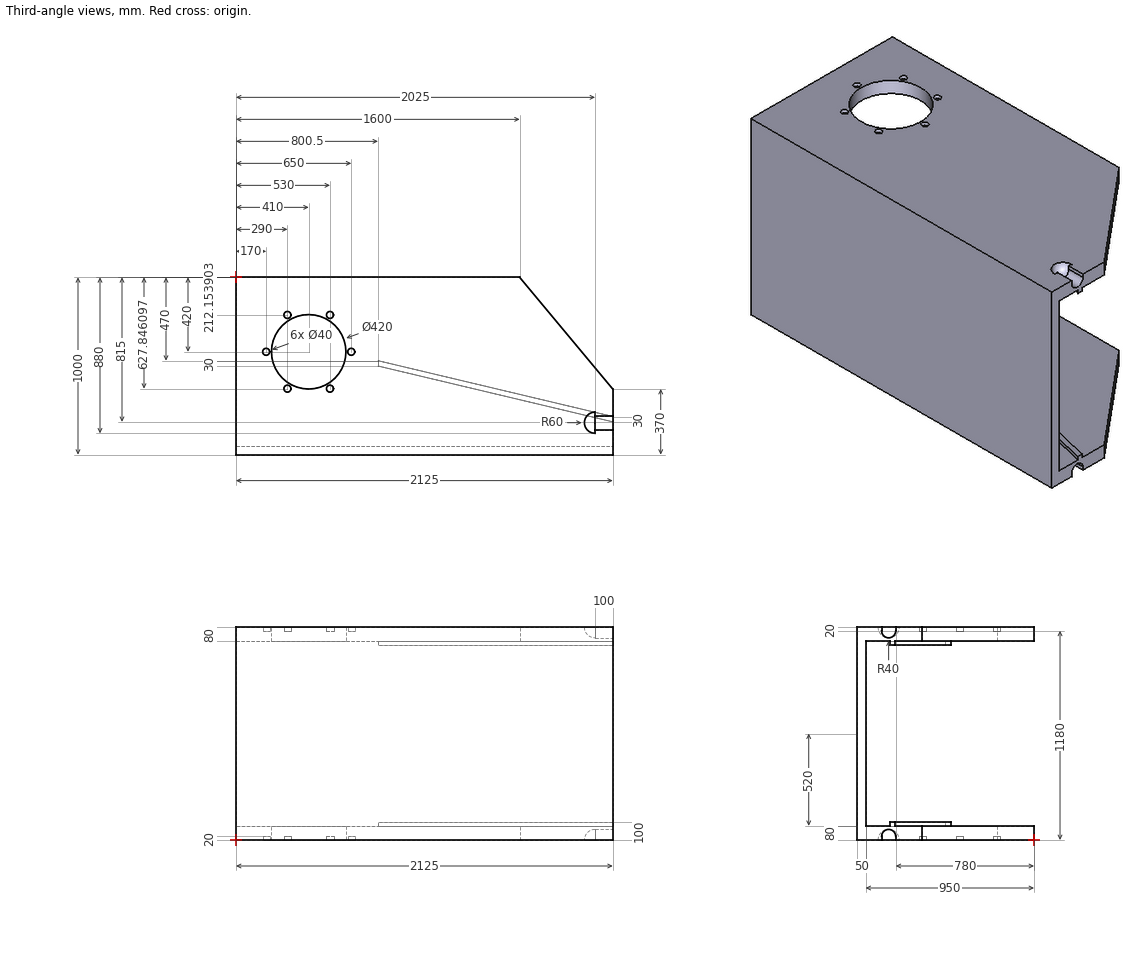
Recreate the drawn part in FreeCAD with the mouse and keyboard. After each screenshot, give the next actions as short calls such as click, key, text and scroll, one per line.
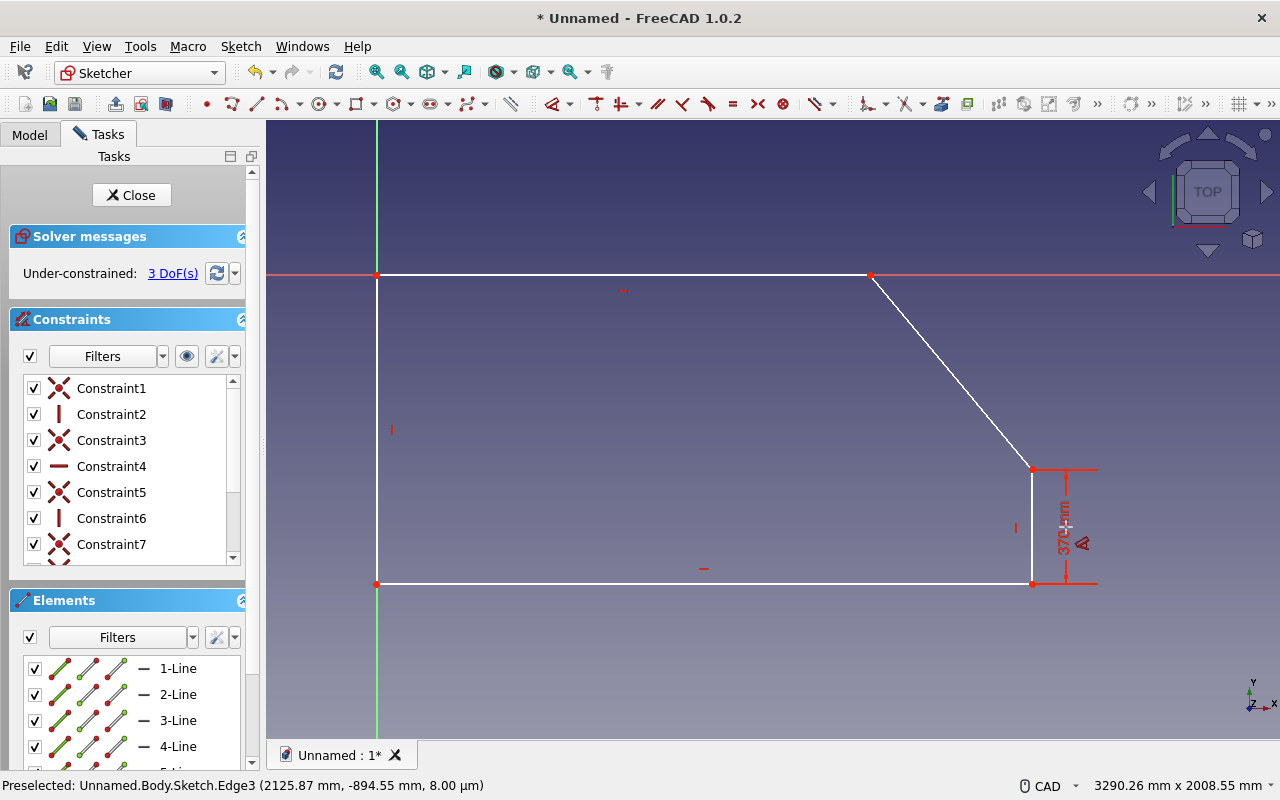
click(377, 368)
click(343, 430)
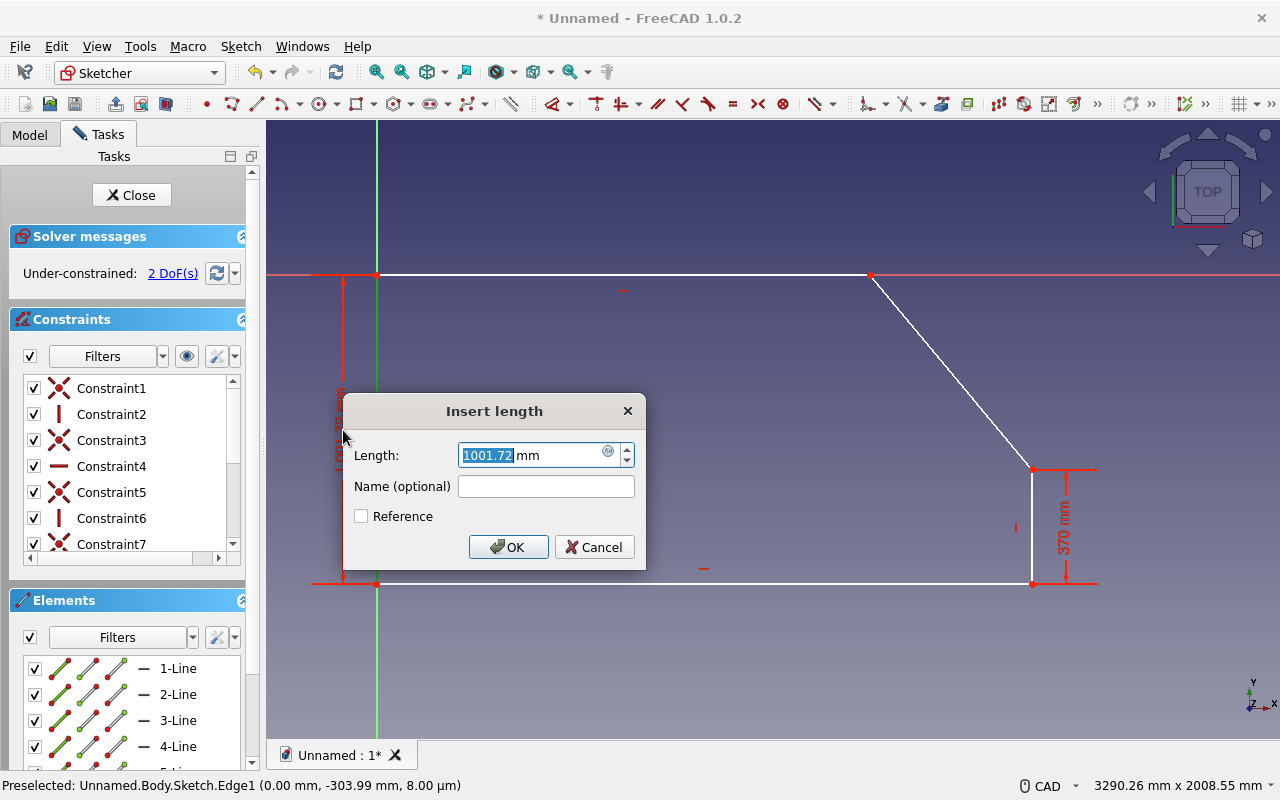
text(1000)
key(Return)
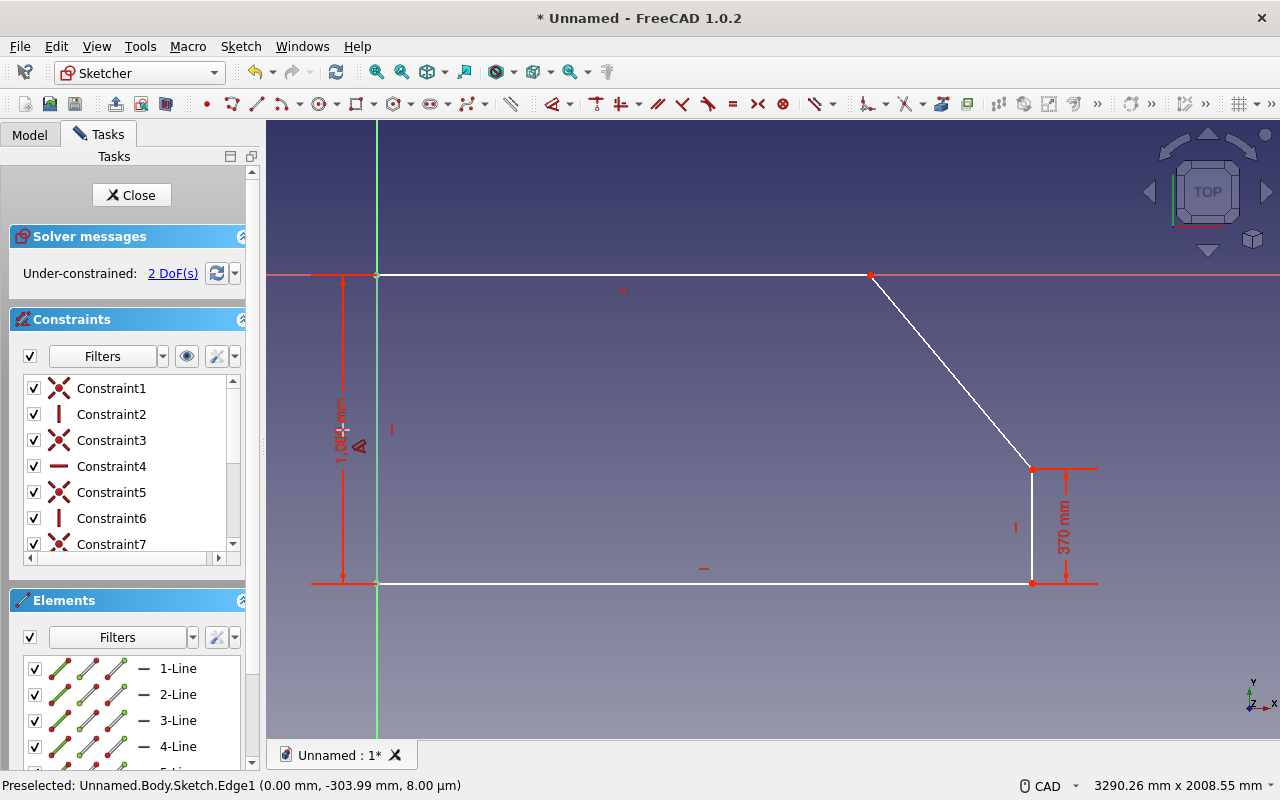
click(573, 583)
click(704, 617)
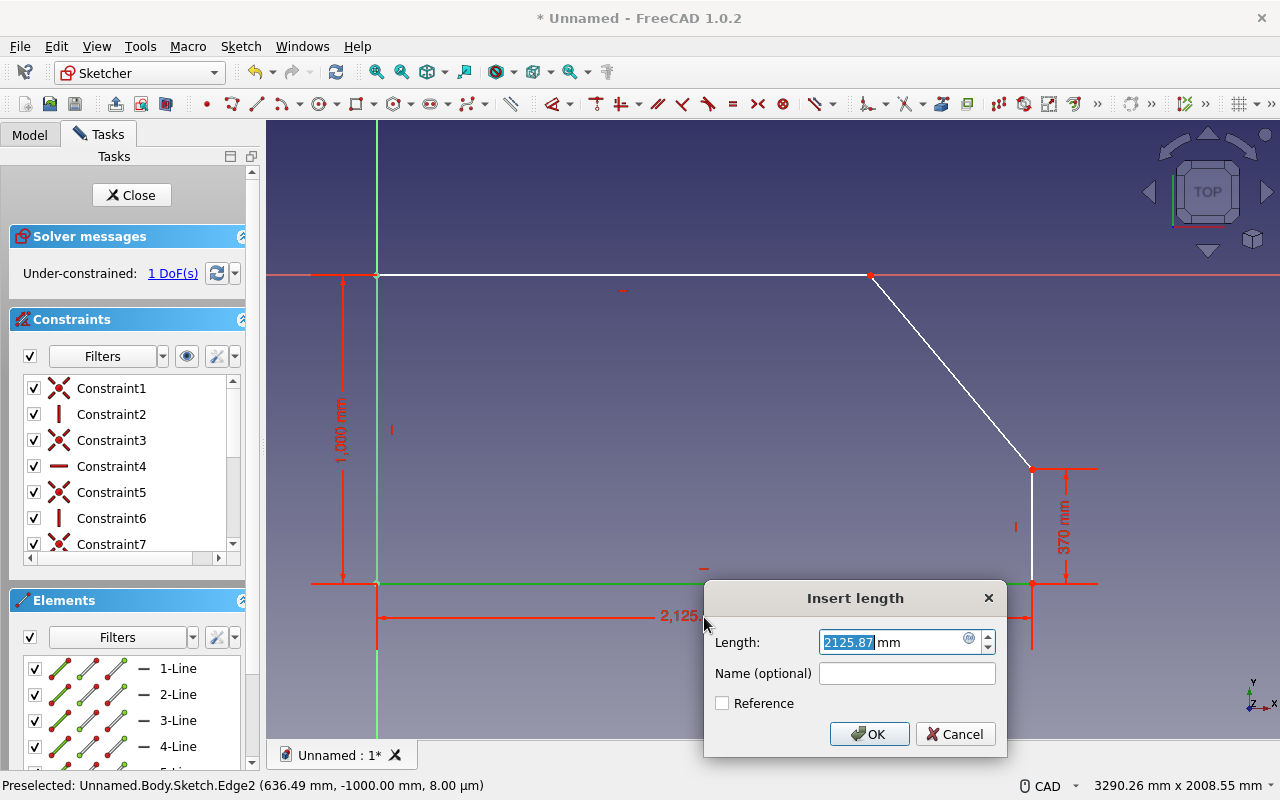
text(2125)
key(Return)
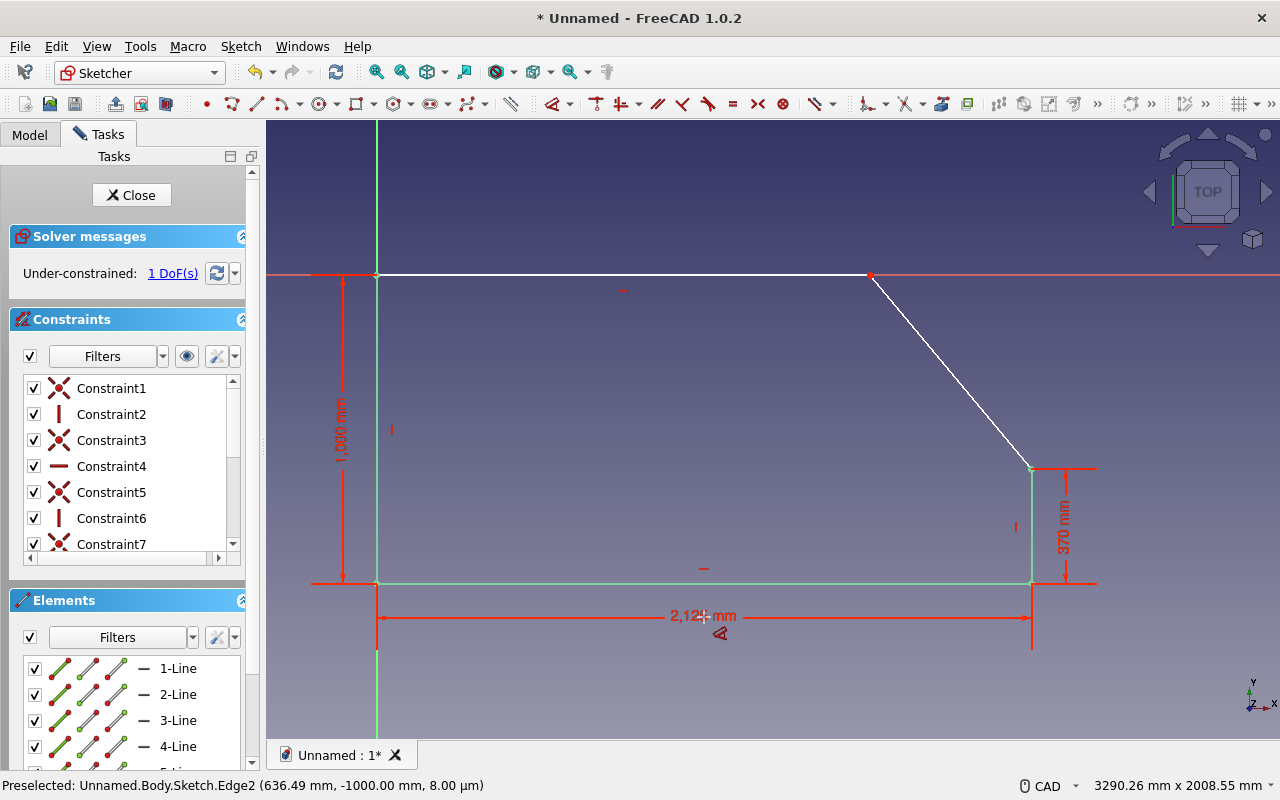
click(722, 275)
click(623, 241)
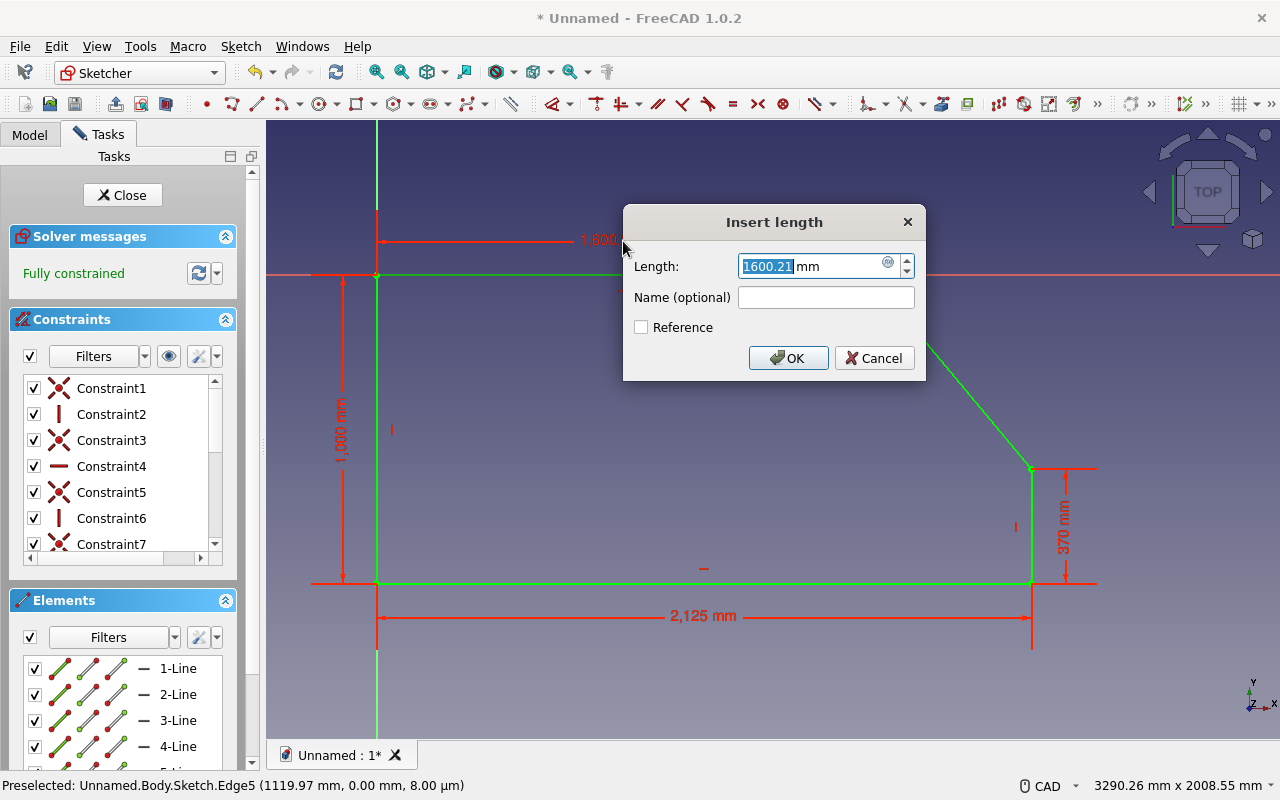
text(1600)
key(Return)
key(Escape)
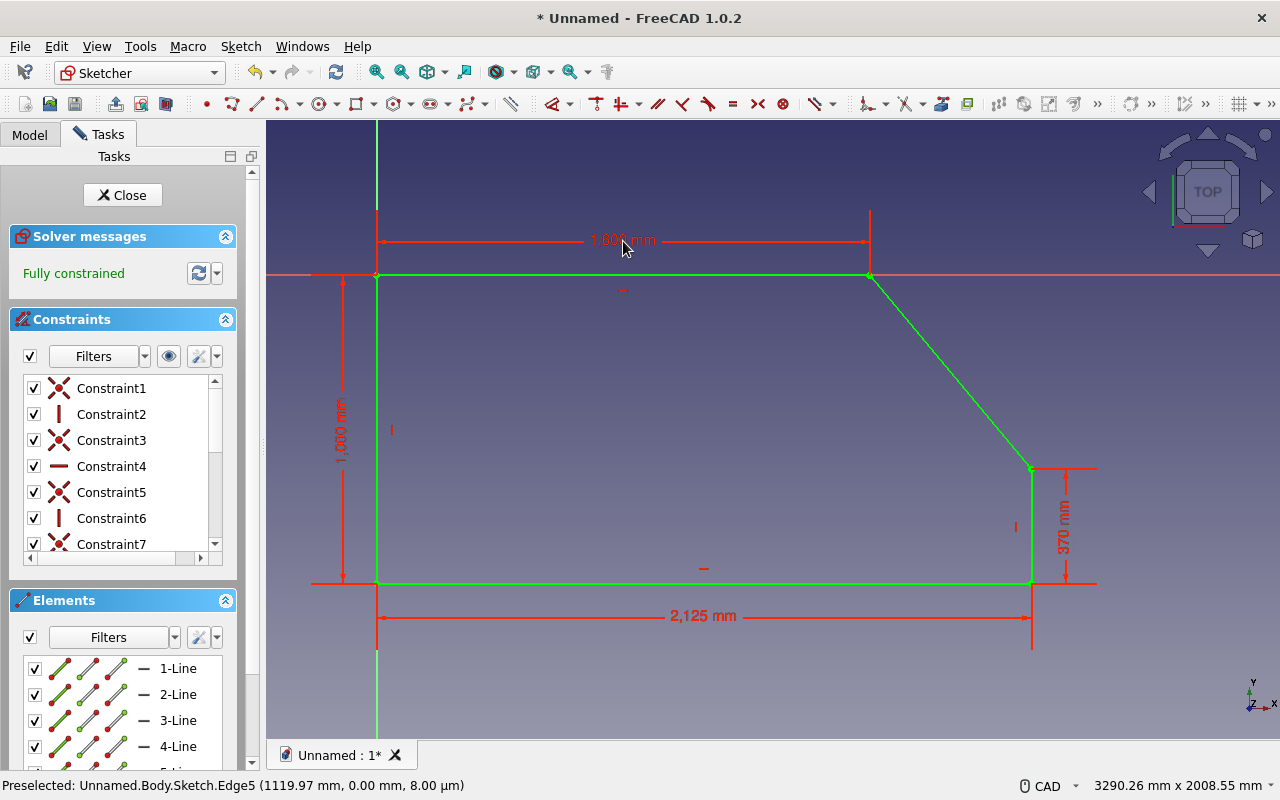
click(123, 195)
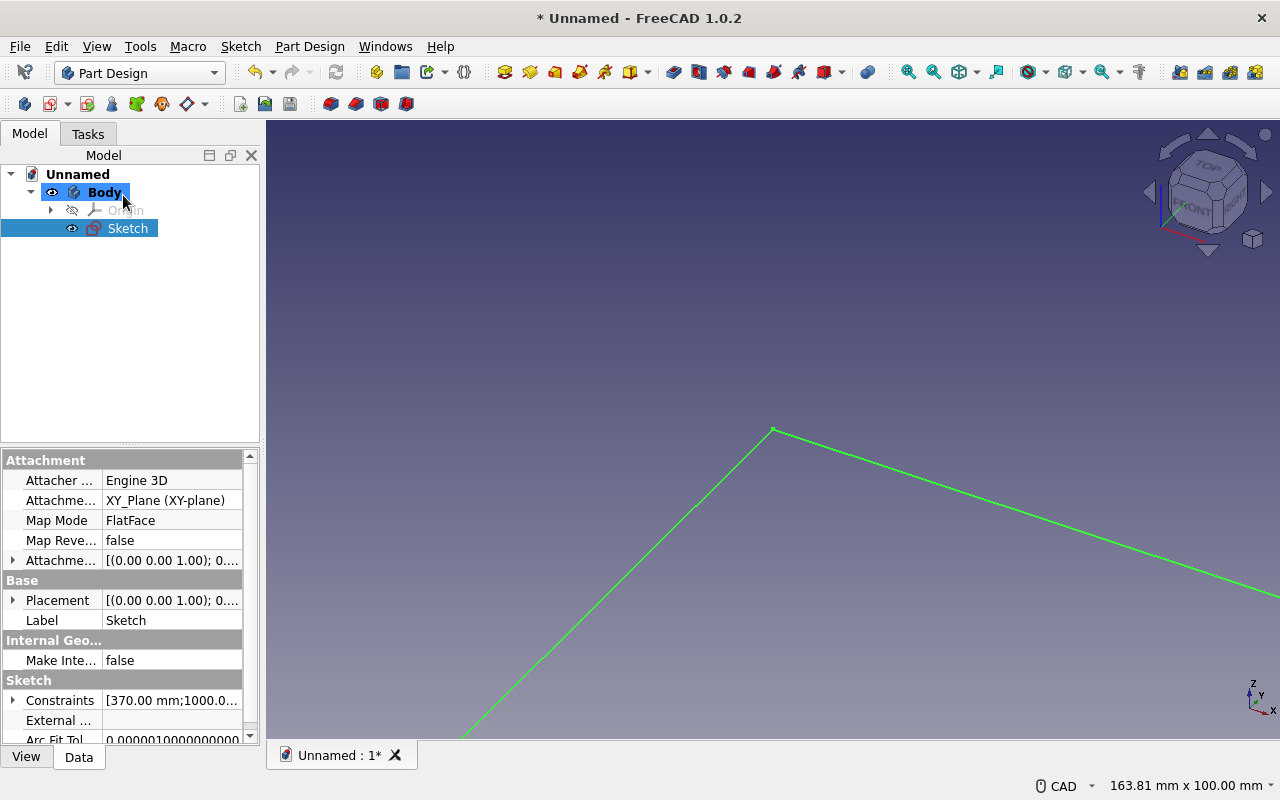
click(505, 72)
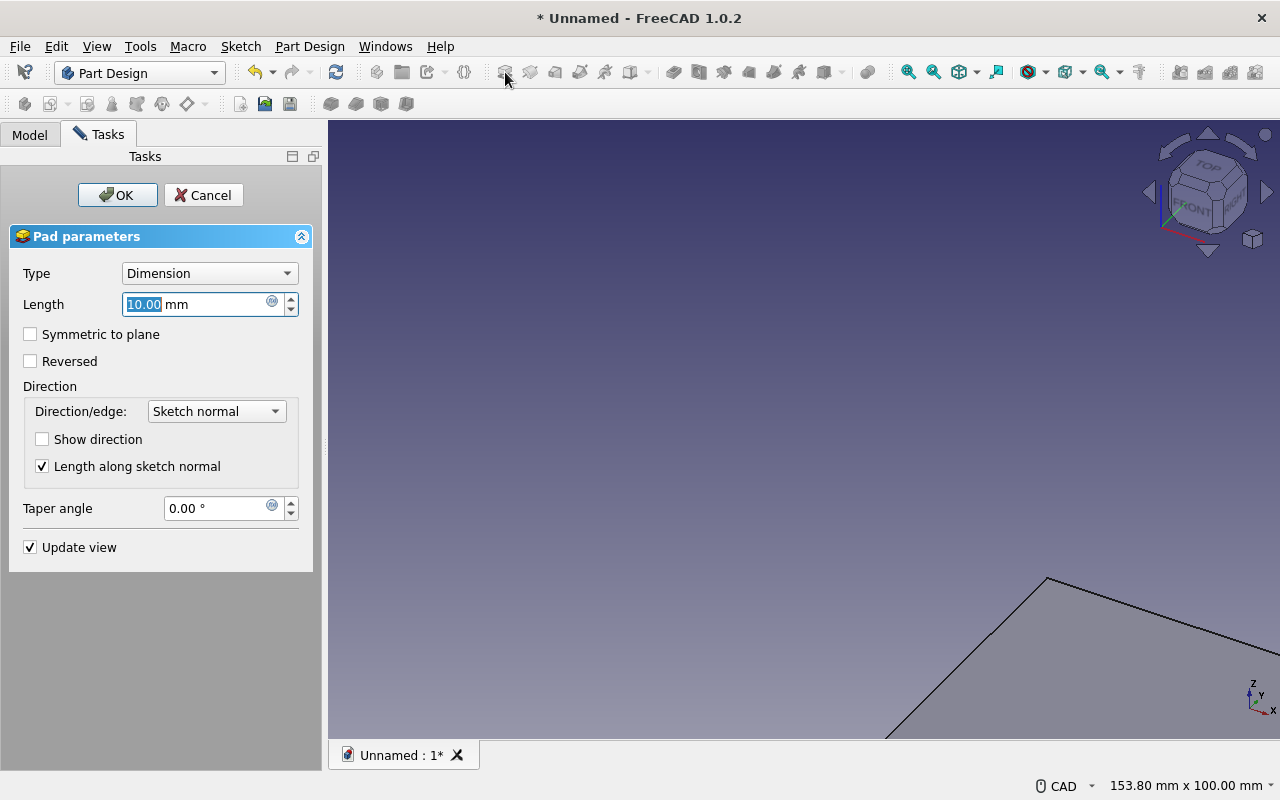
text(80)
key(Tab)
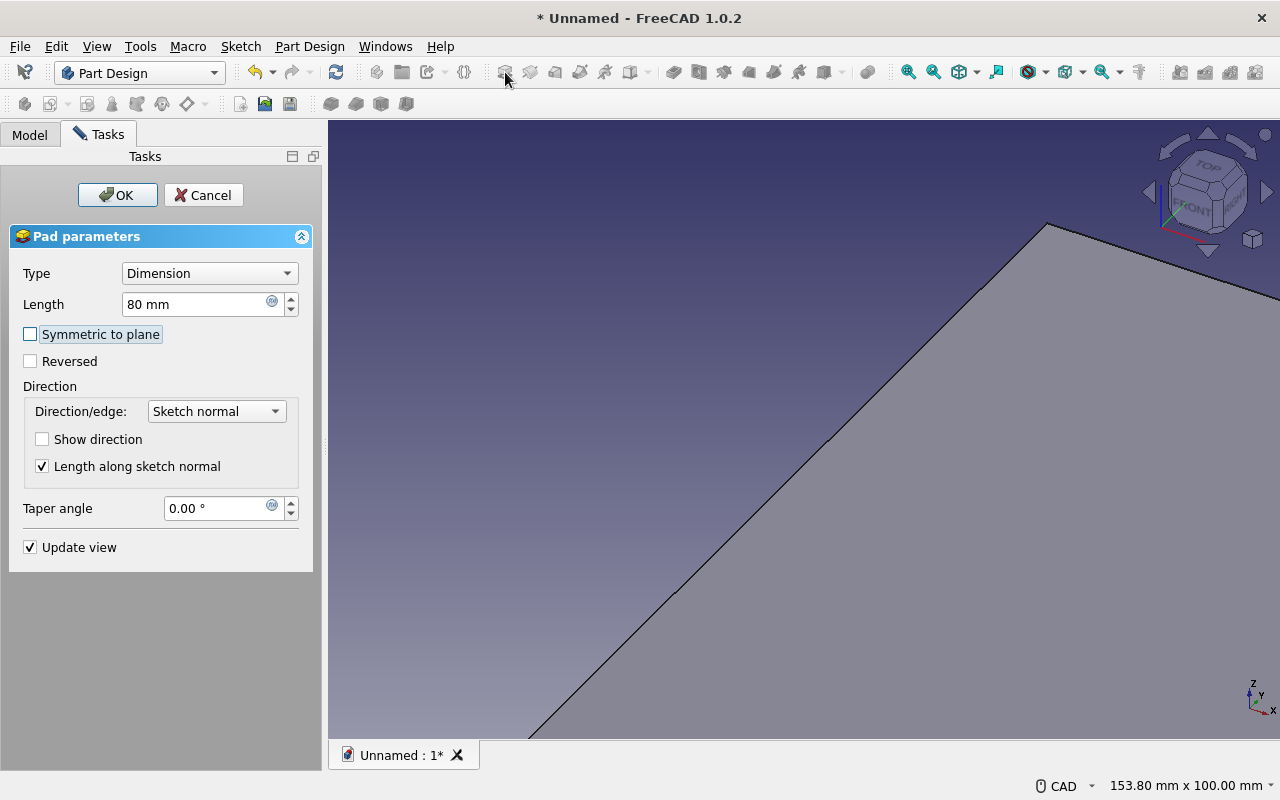
click(118, 195)